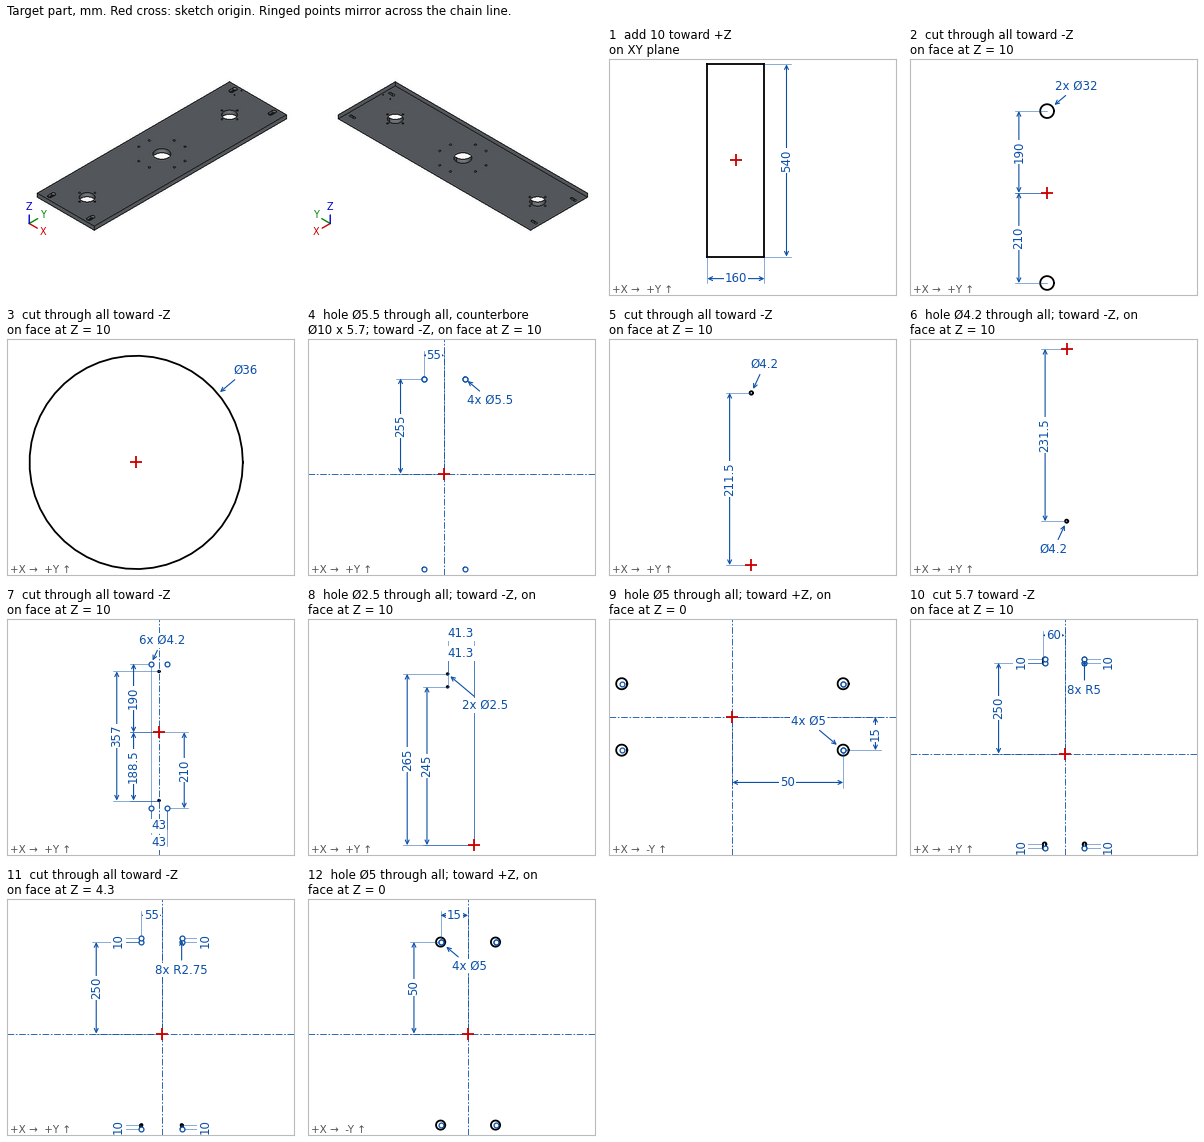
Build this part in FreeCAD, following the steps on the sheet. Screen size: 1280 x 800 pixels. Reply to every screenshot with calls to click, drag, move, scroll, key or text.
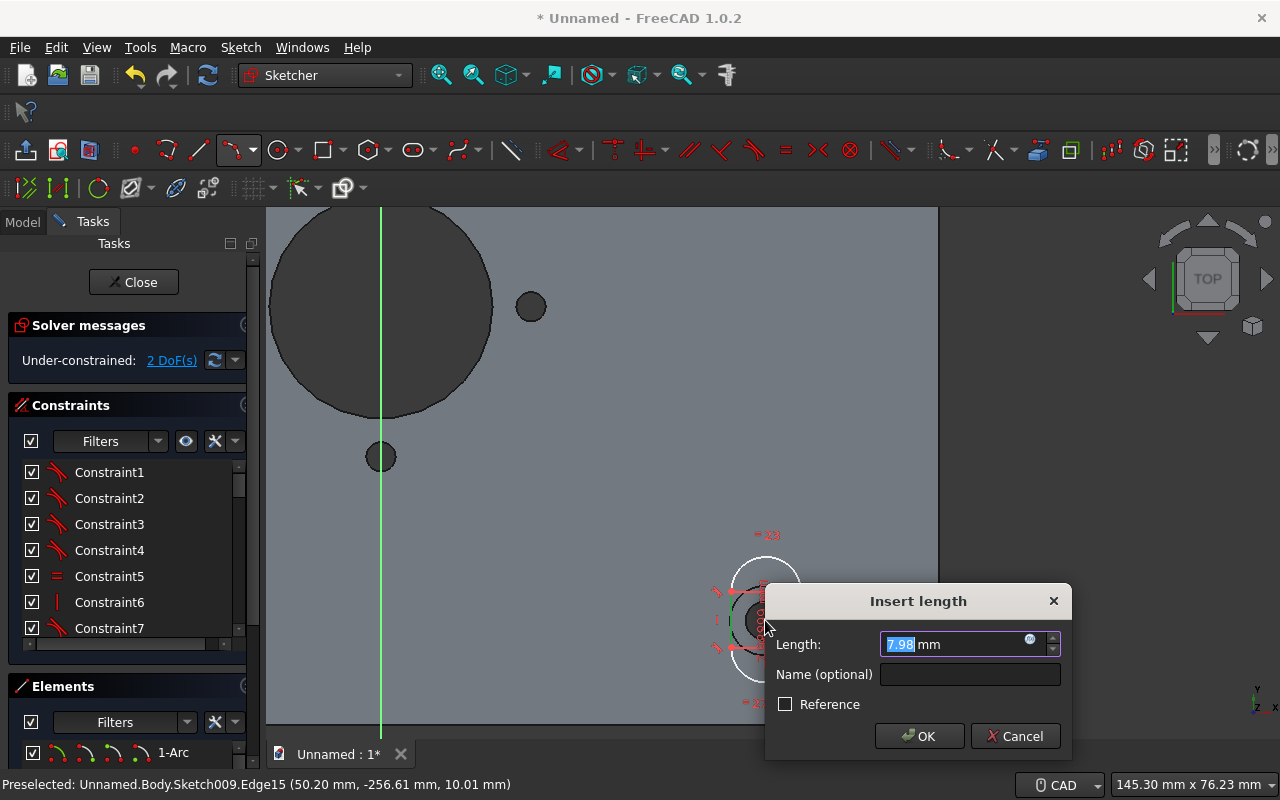
text(10)
key(Return)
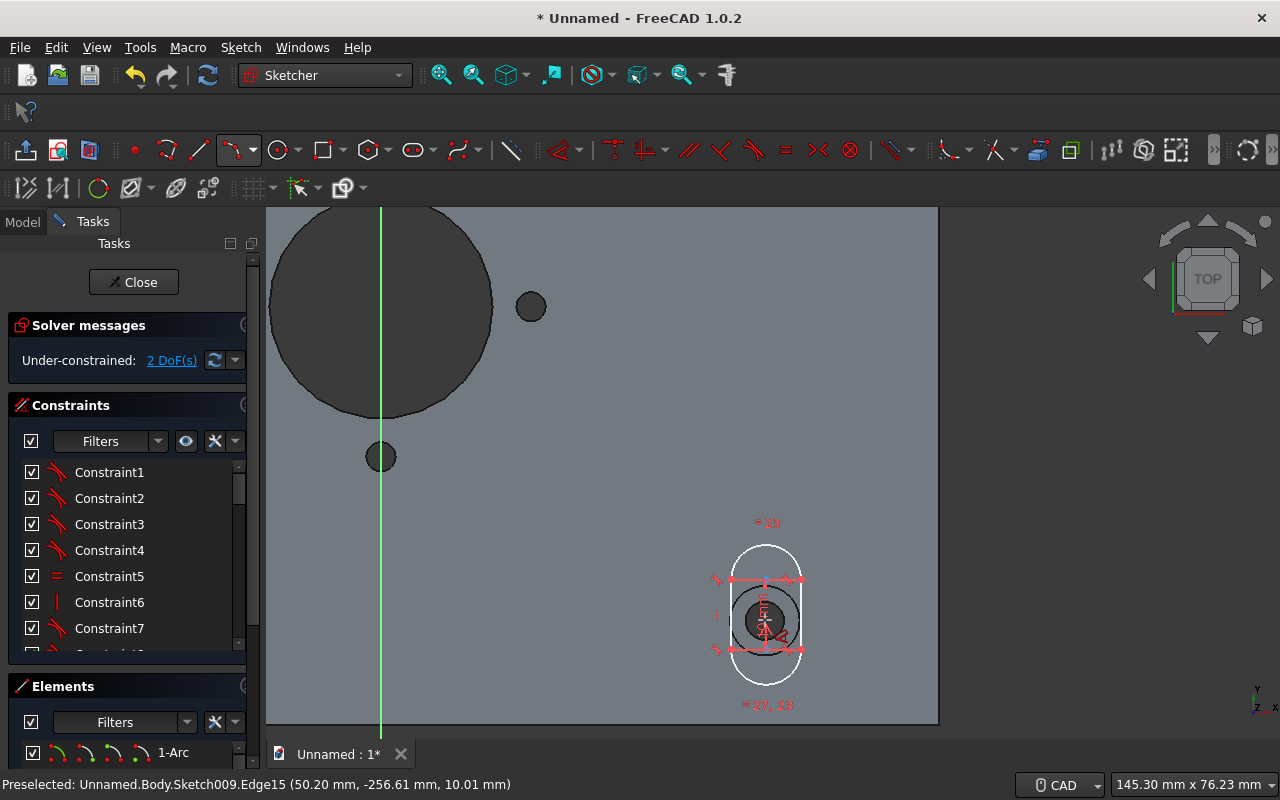
scroll(737, 636, down, 12)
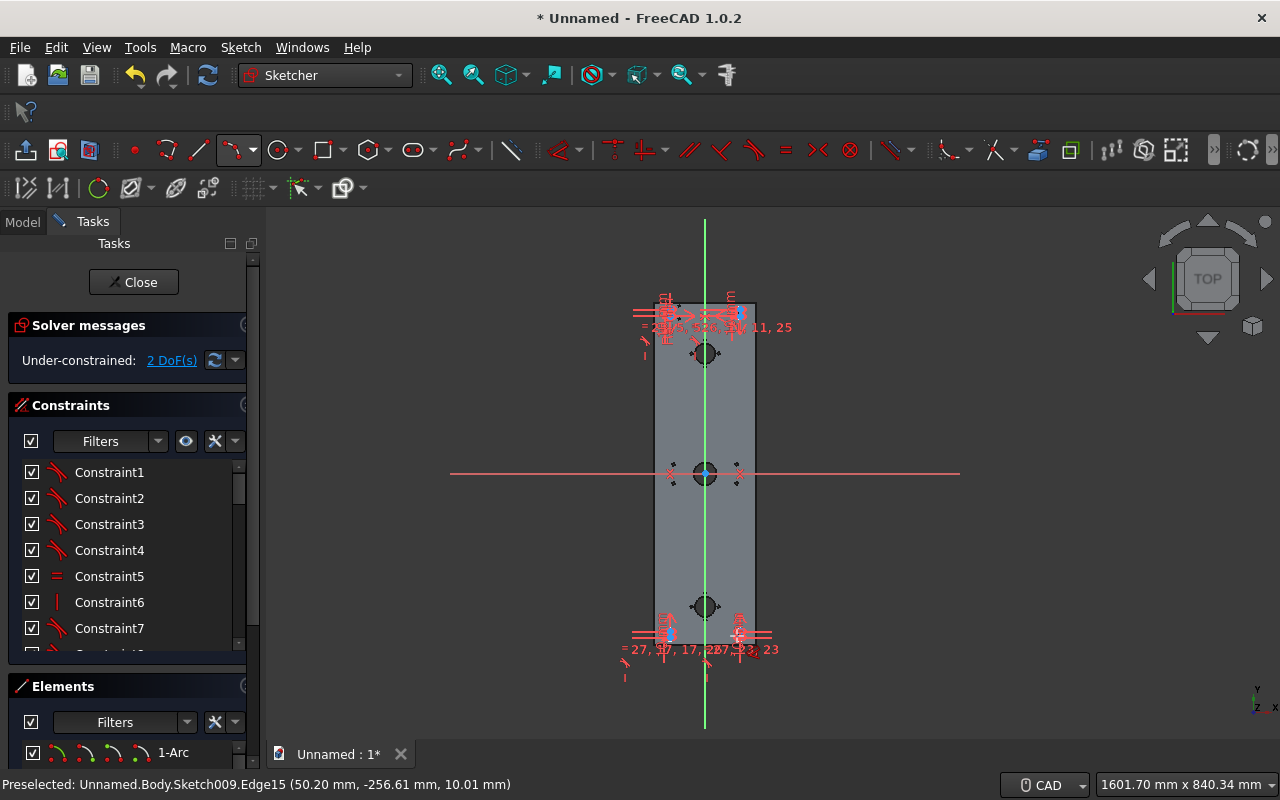
scroll(667, 316, up, 7)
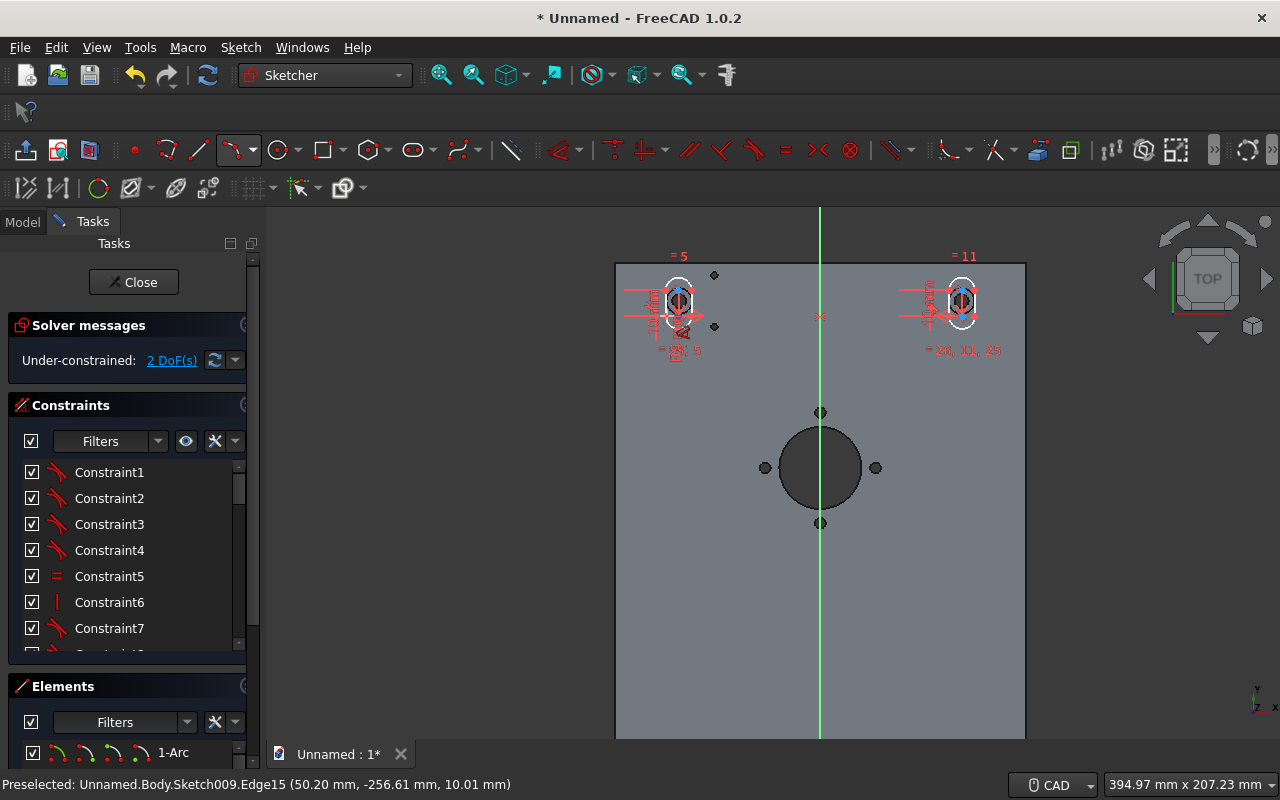
click(666, 316)
click(743, 282)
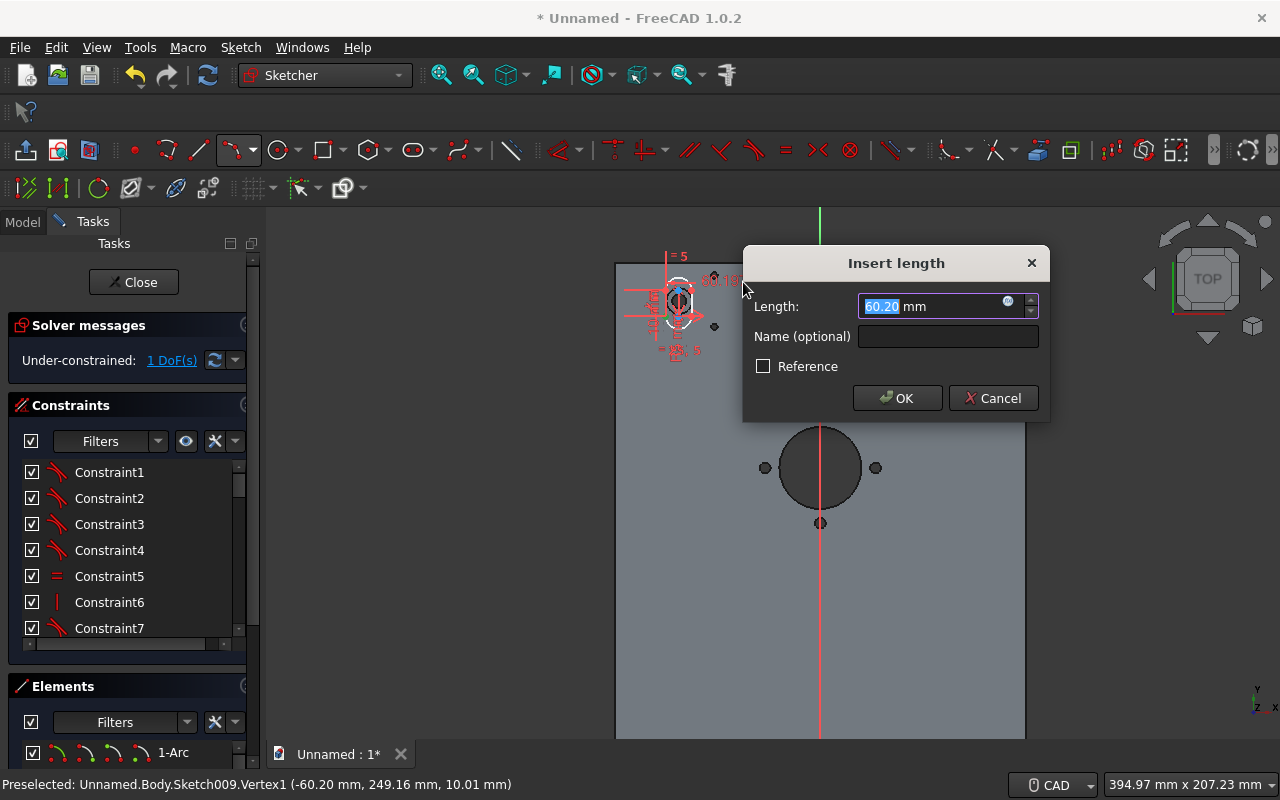
text(60)
key(Return)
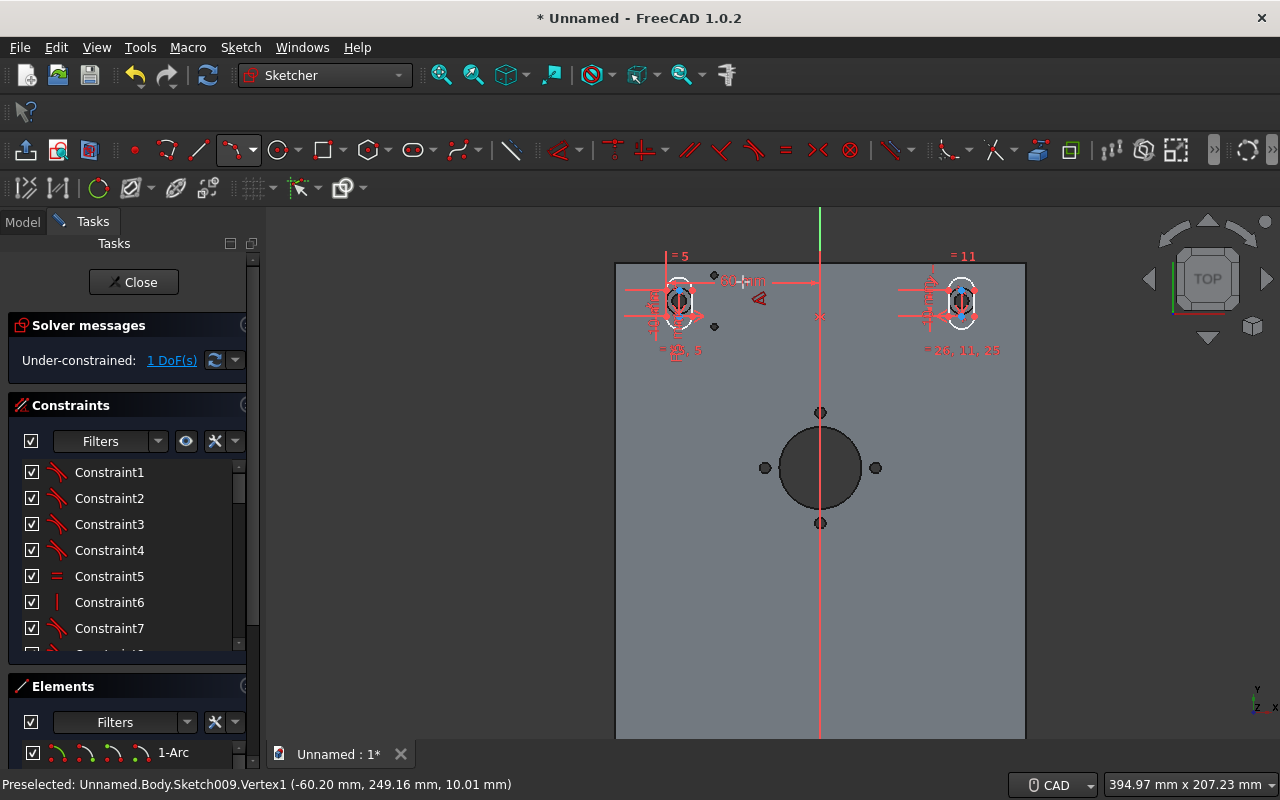
click(666, 316)
click(632, 514)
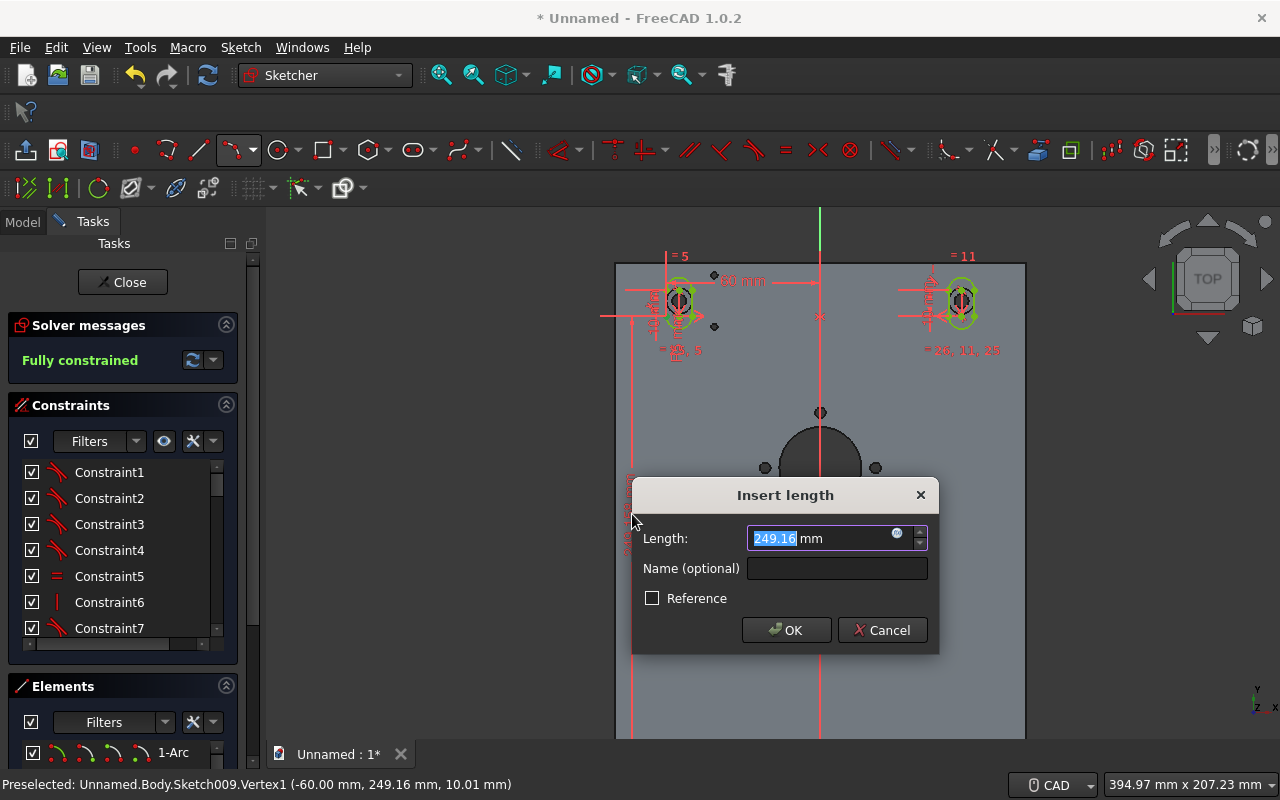
text(250)
key(Return)
key(Escape)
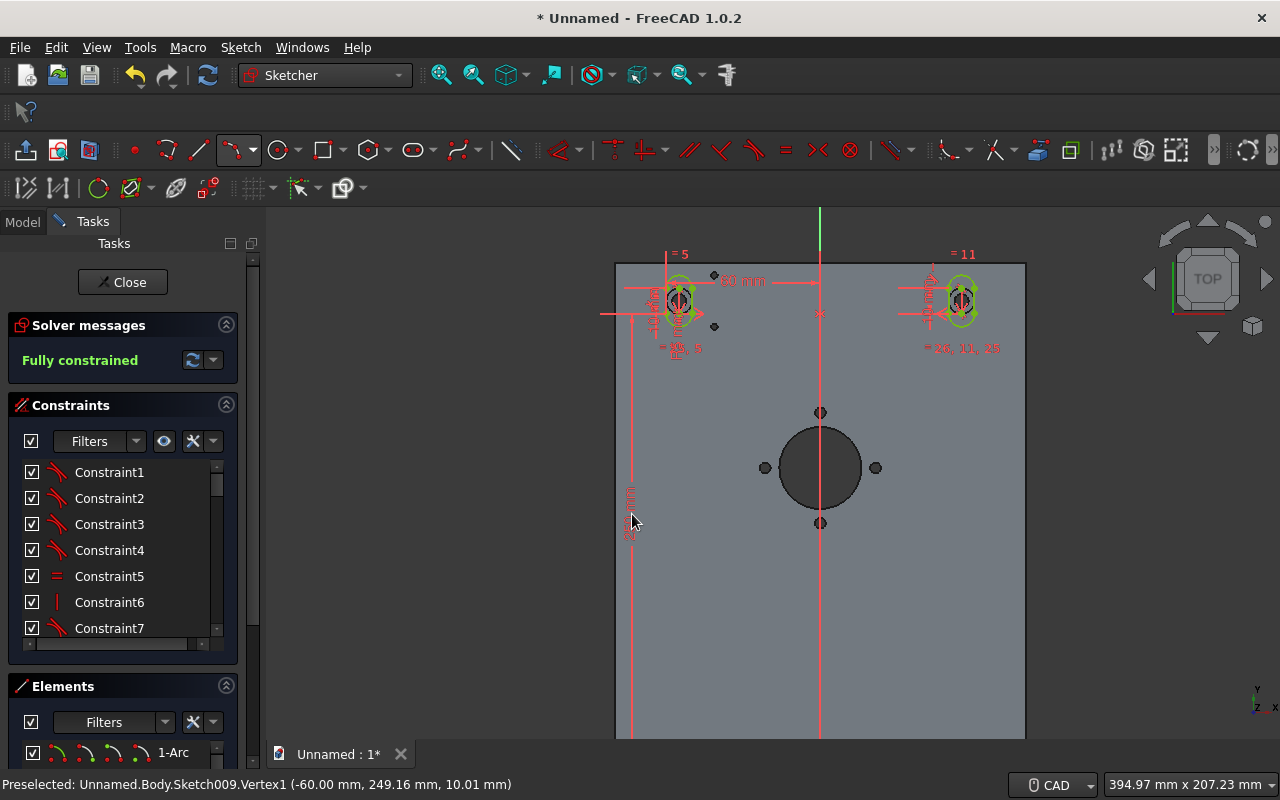
click(123, 282)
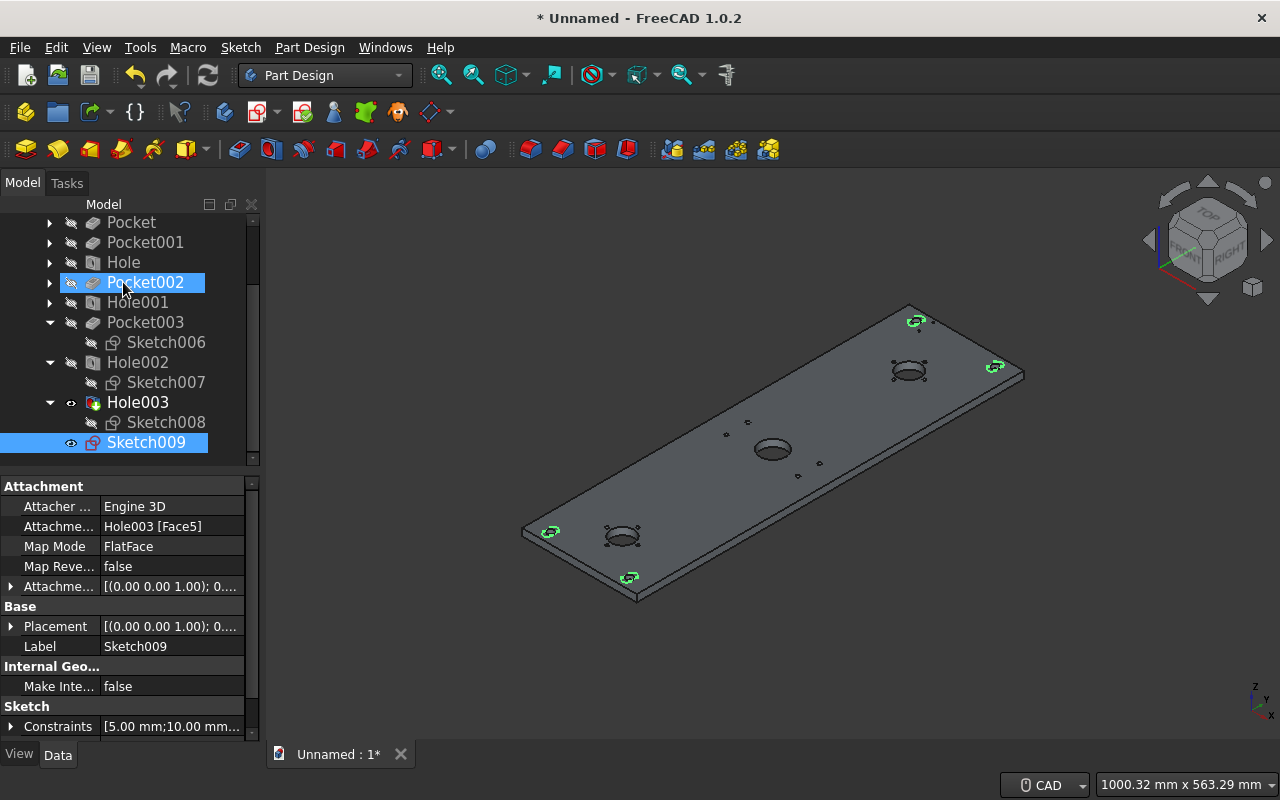
click(240, 150)